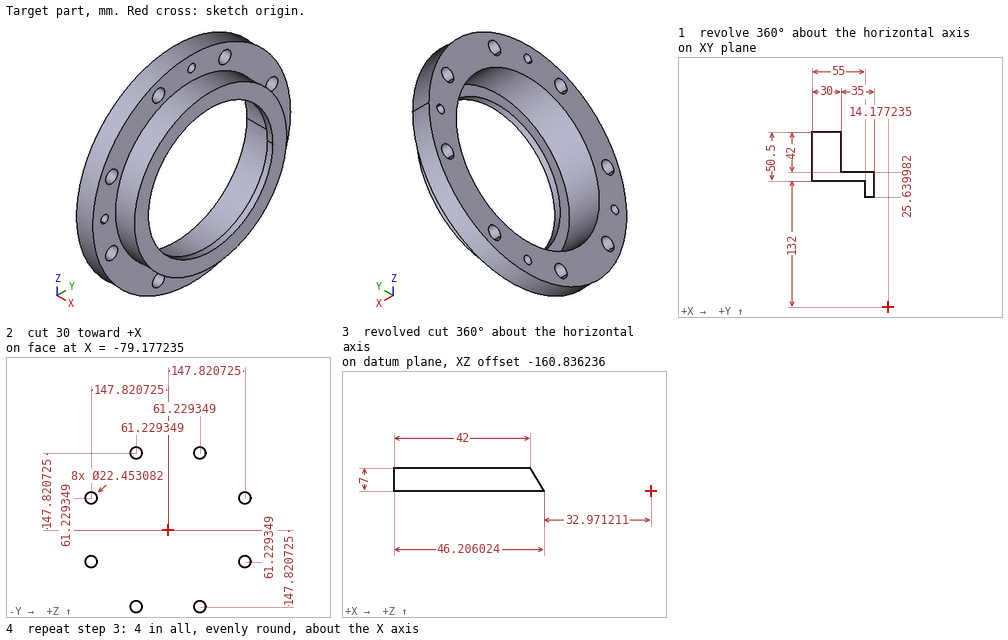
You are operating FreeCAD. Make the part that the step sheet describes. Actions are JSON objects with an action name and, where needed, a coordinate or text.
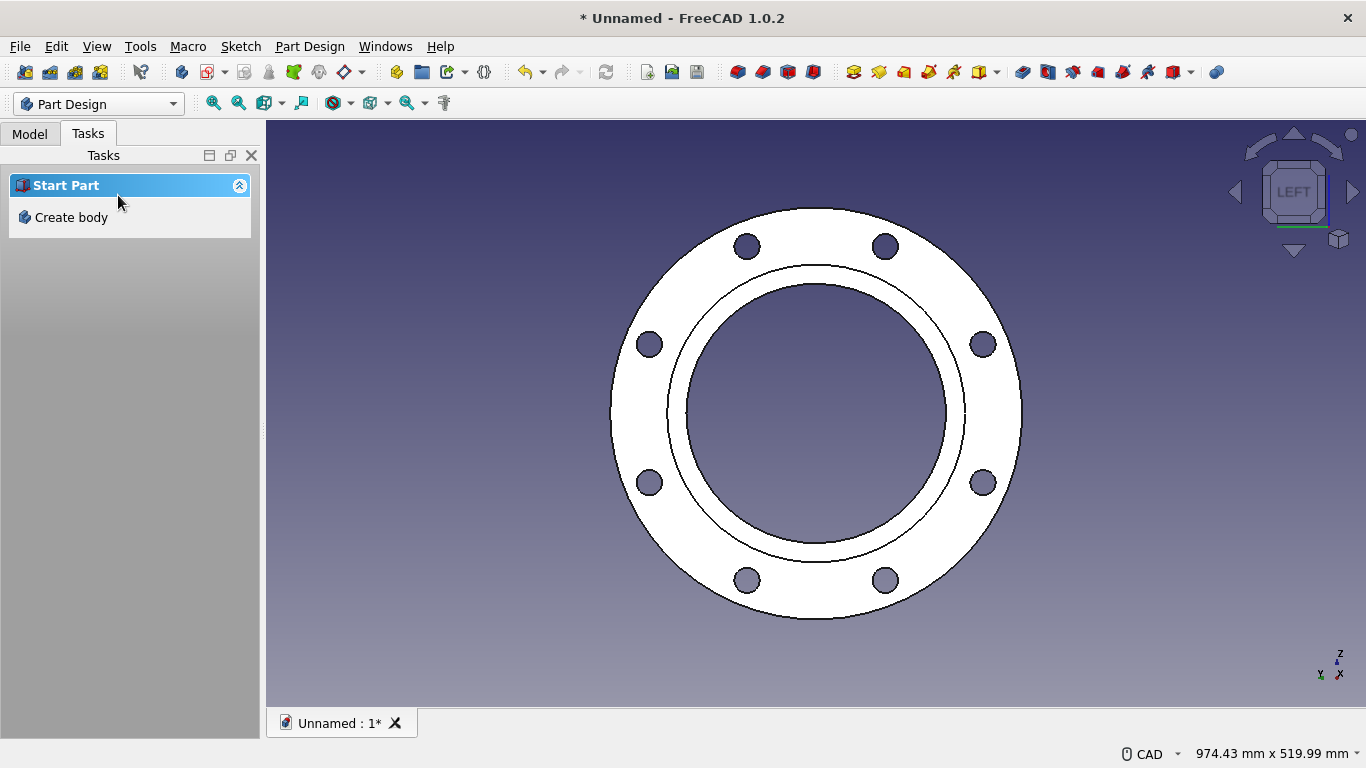
{"action": "left_click", "coordinate": [30, 134]}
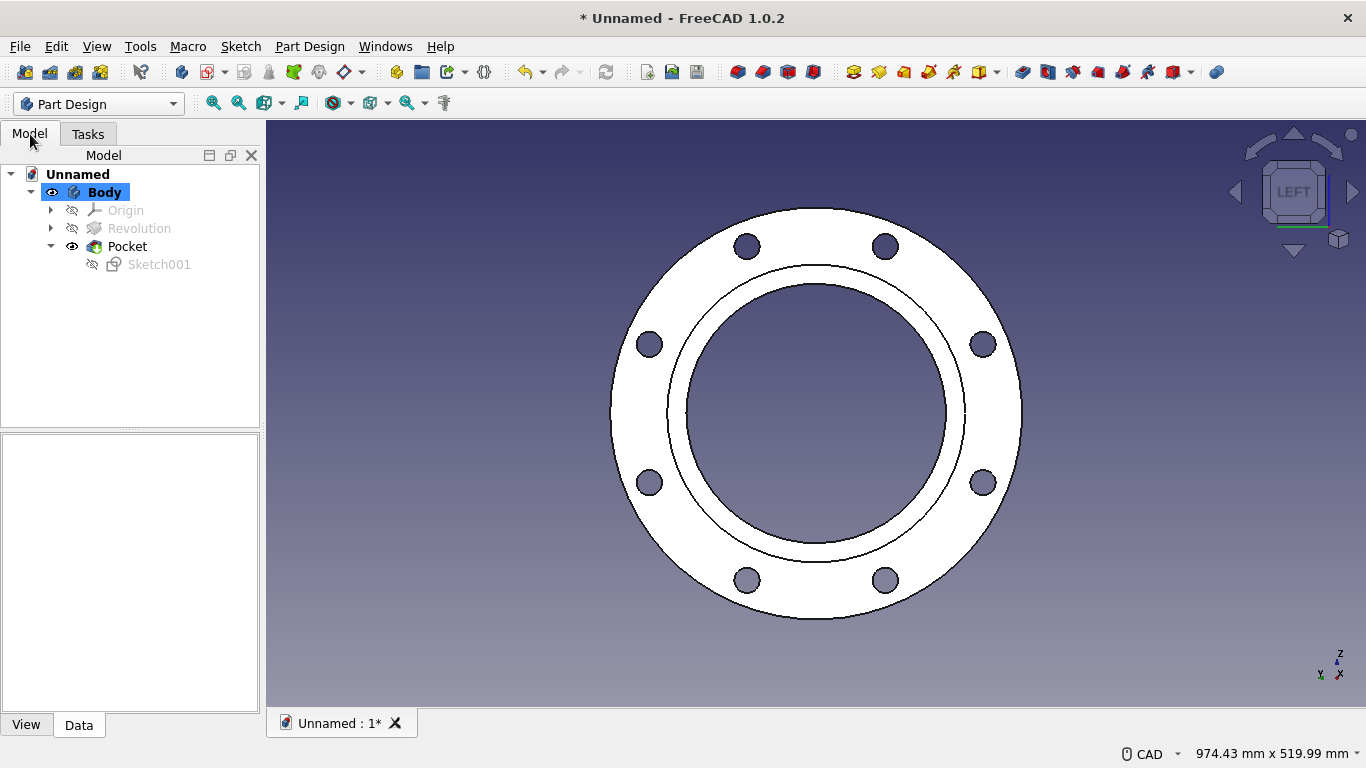
{"action": "left_click", "coordinate": [51, 210]}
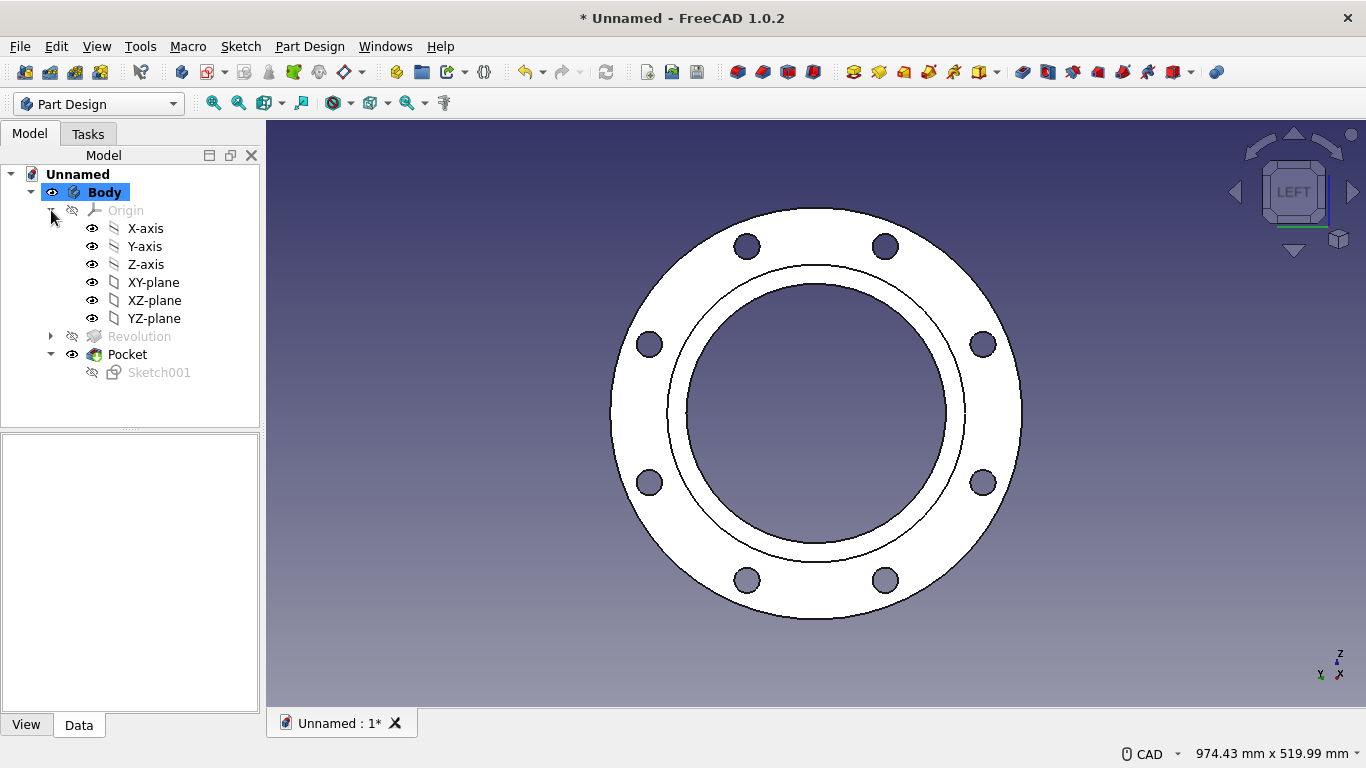
{"action": "left_click", "coordinate": [137, 300]}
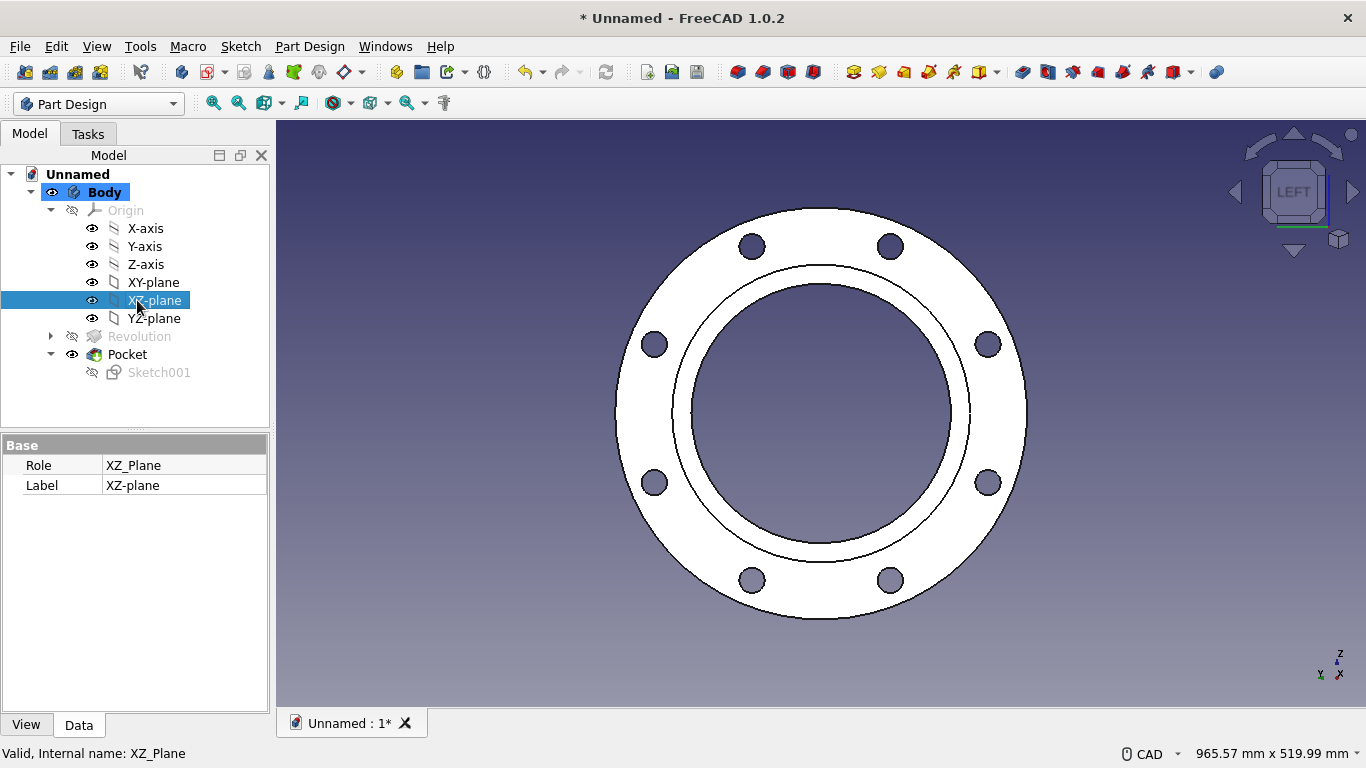
{"action": "left_click", "coordinate": [344, 72]}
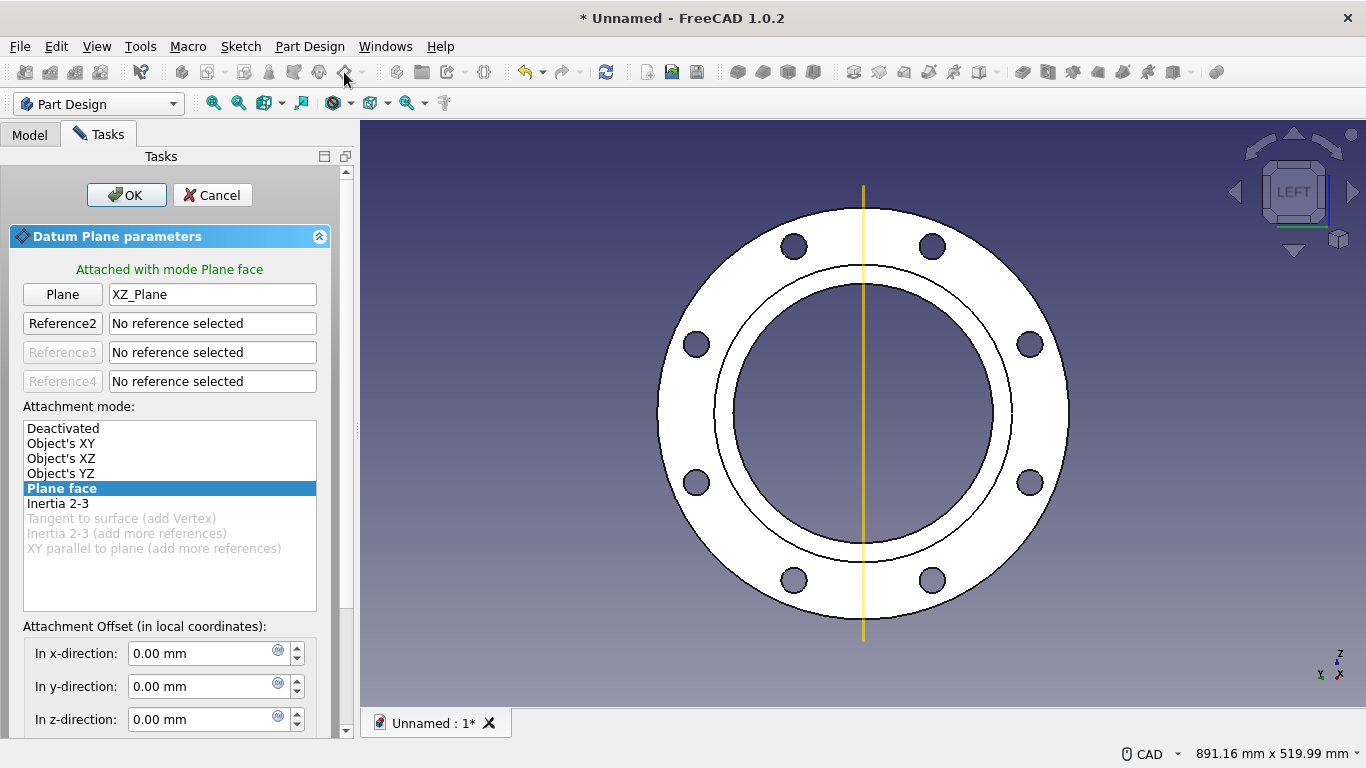
{"action": "triple_click", "coordinate": [210, 720]}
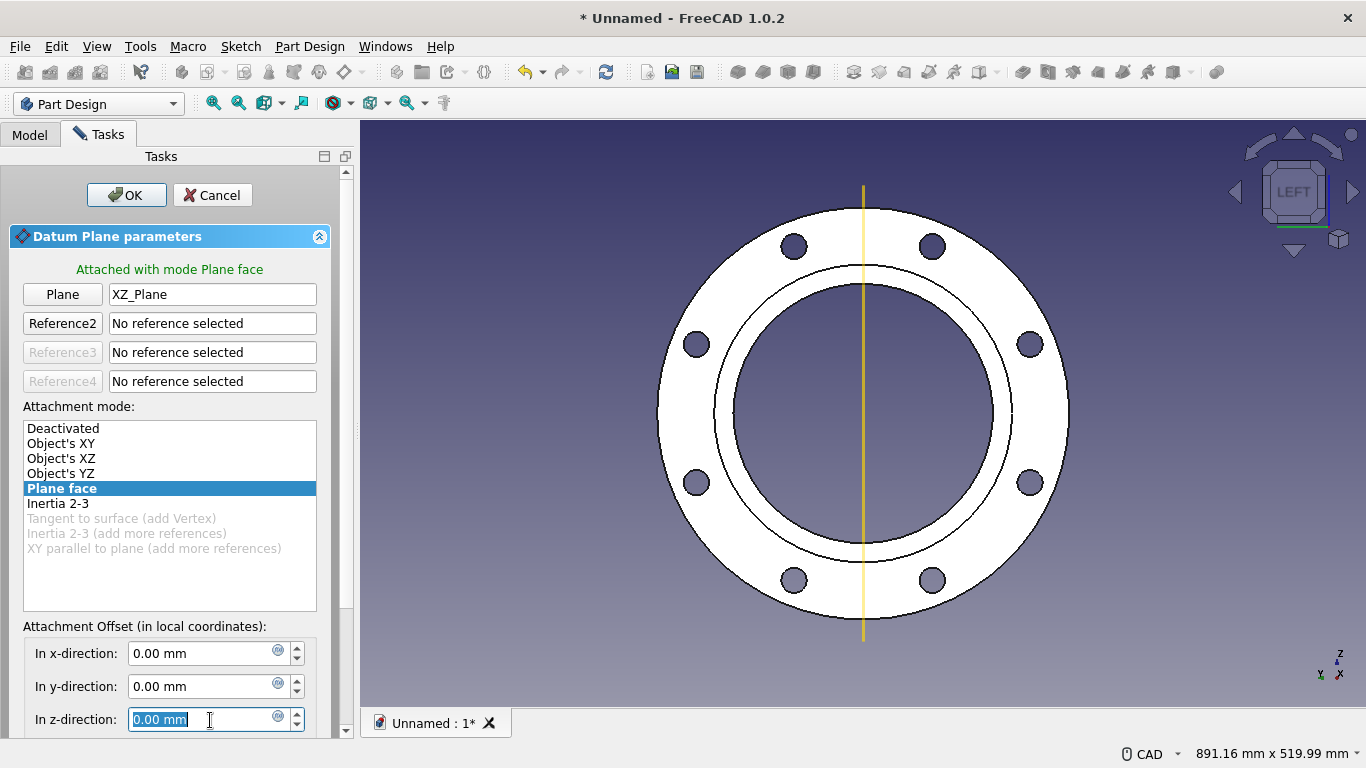
{"action": "type", "text": "-160.836236"}
{"action": "key", "text": "Tab"}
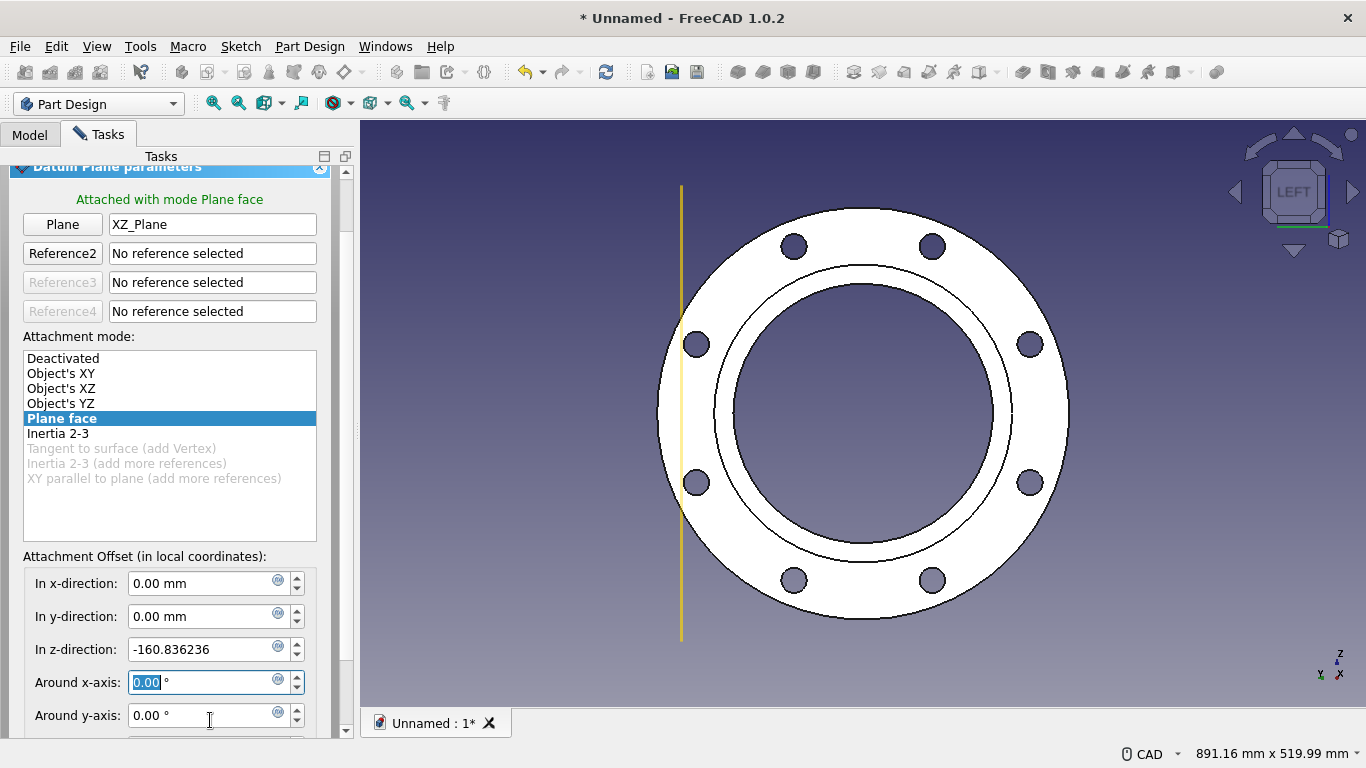
{"action": "scroll", "coordinate": [346, 452], "scroll_direction": "up", "scroll_amount": 2}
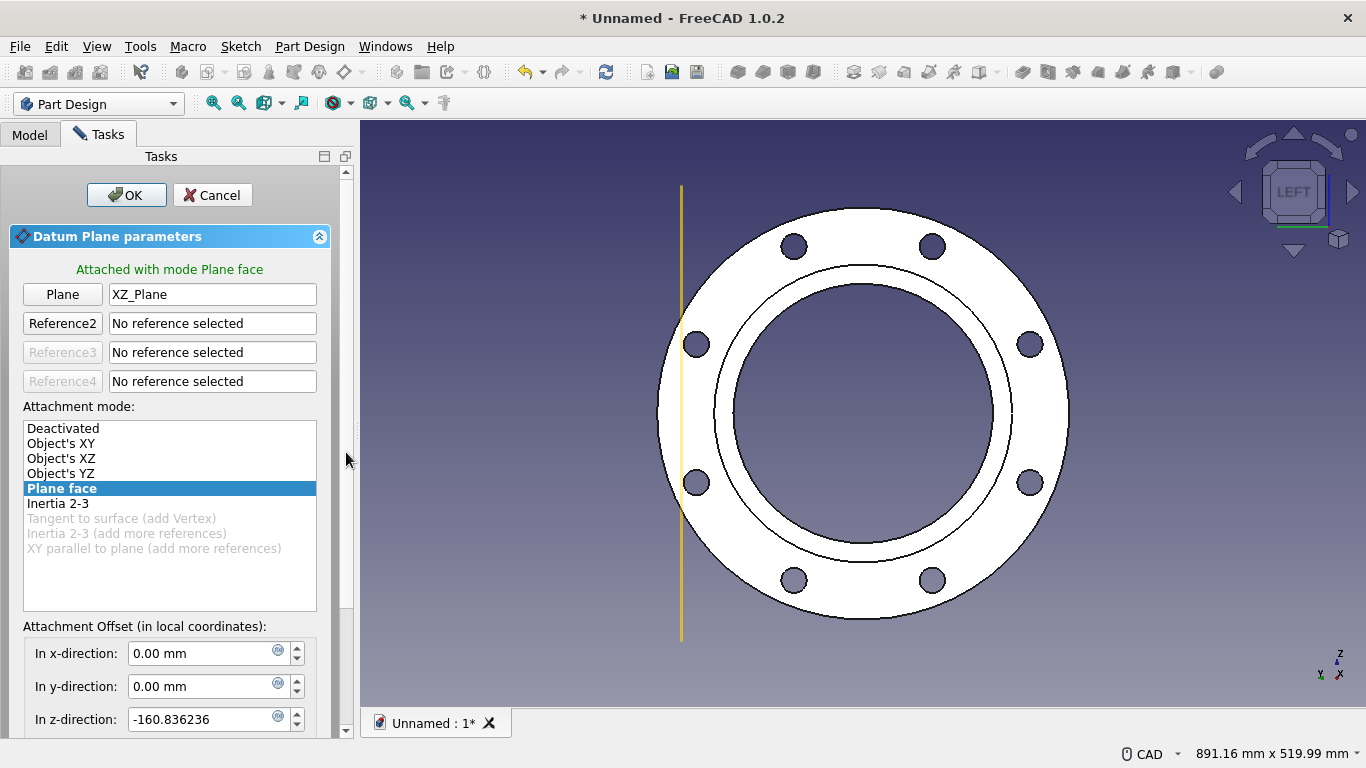
{"action": "left_click", "coordinate": [127, 195]}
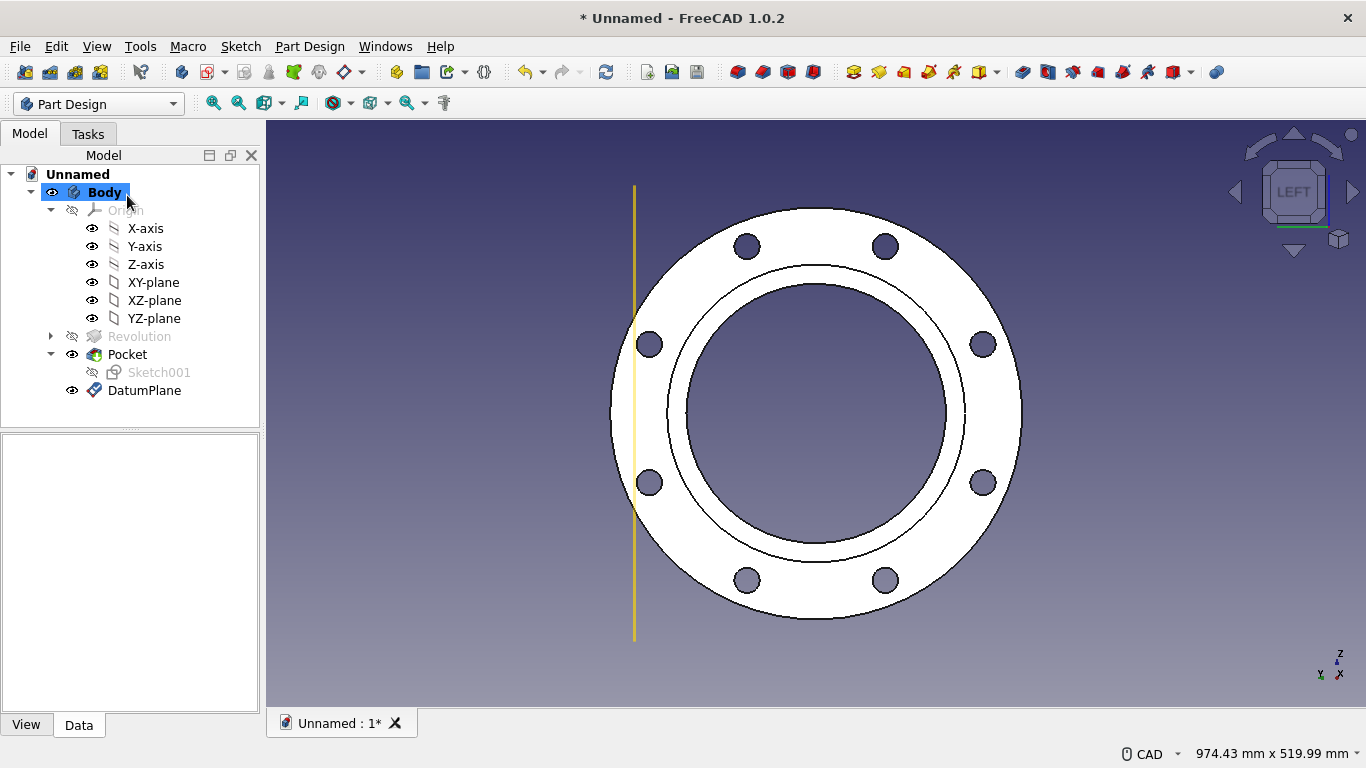
{"action": "left_click", "coordinate": [117, 390]}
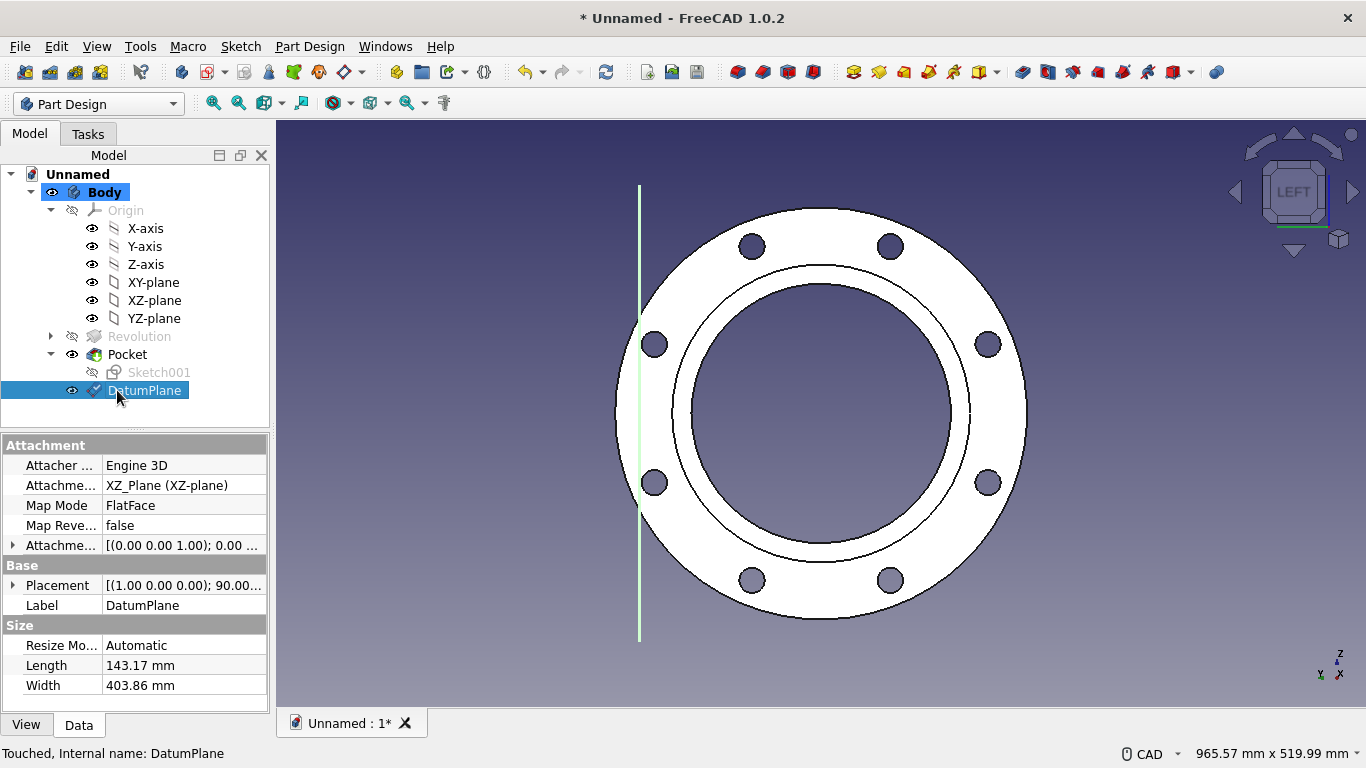
{"action": "left_click", "coordinate": [206, 72]}